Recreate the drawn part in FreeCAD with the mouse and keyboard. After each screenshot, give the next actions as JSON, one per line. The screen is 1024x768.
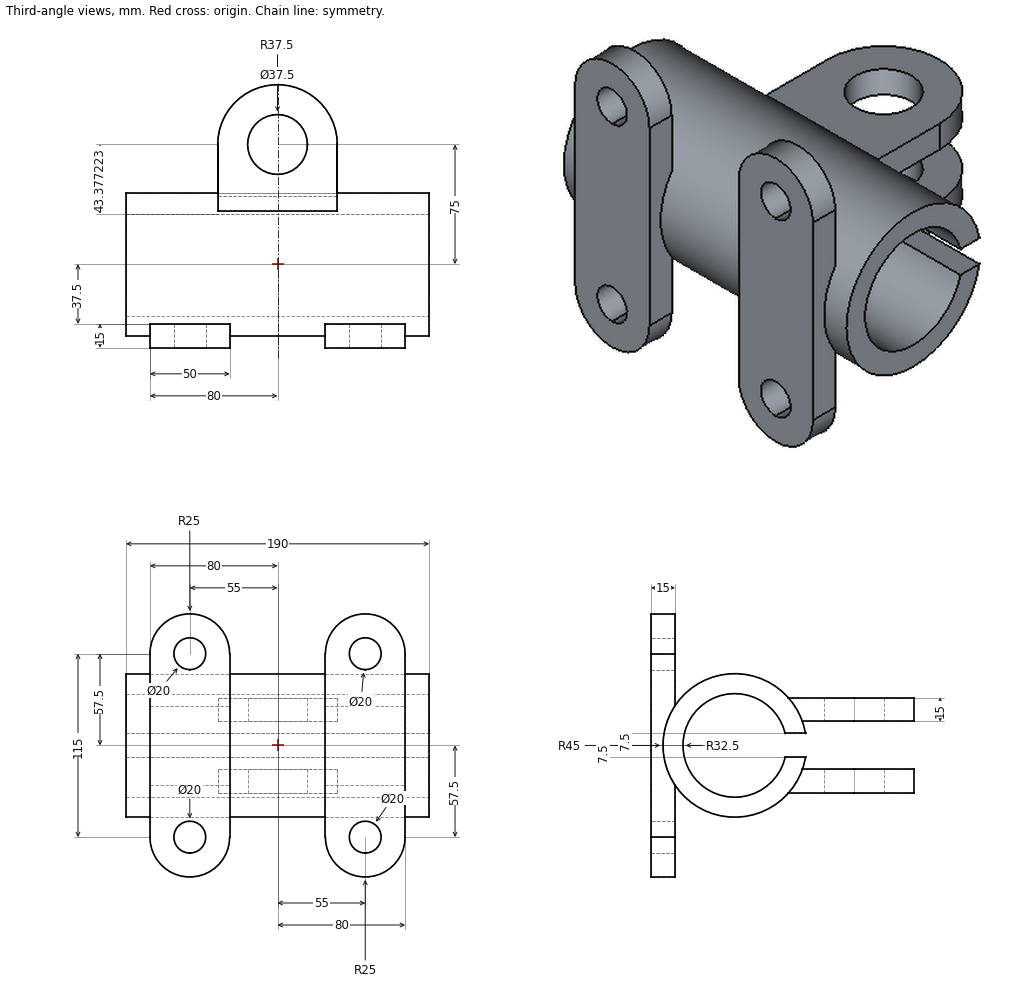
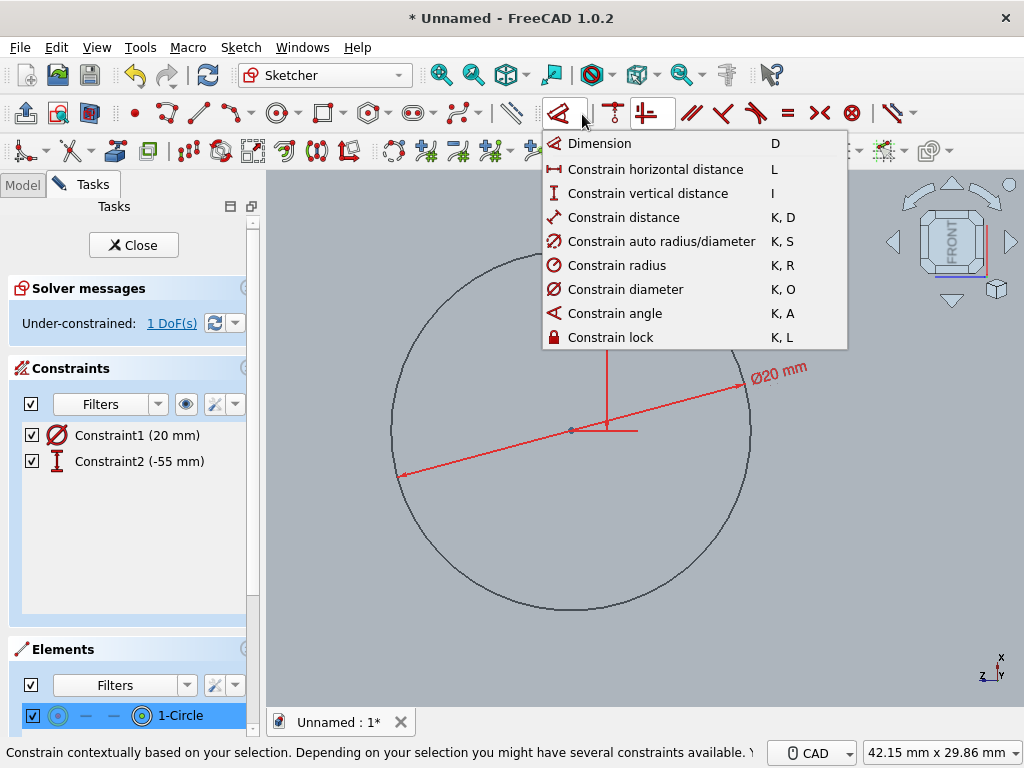
{"action": "left_click", "coordinate": [695, 169]}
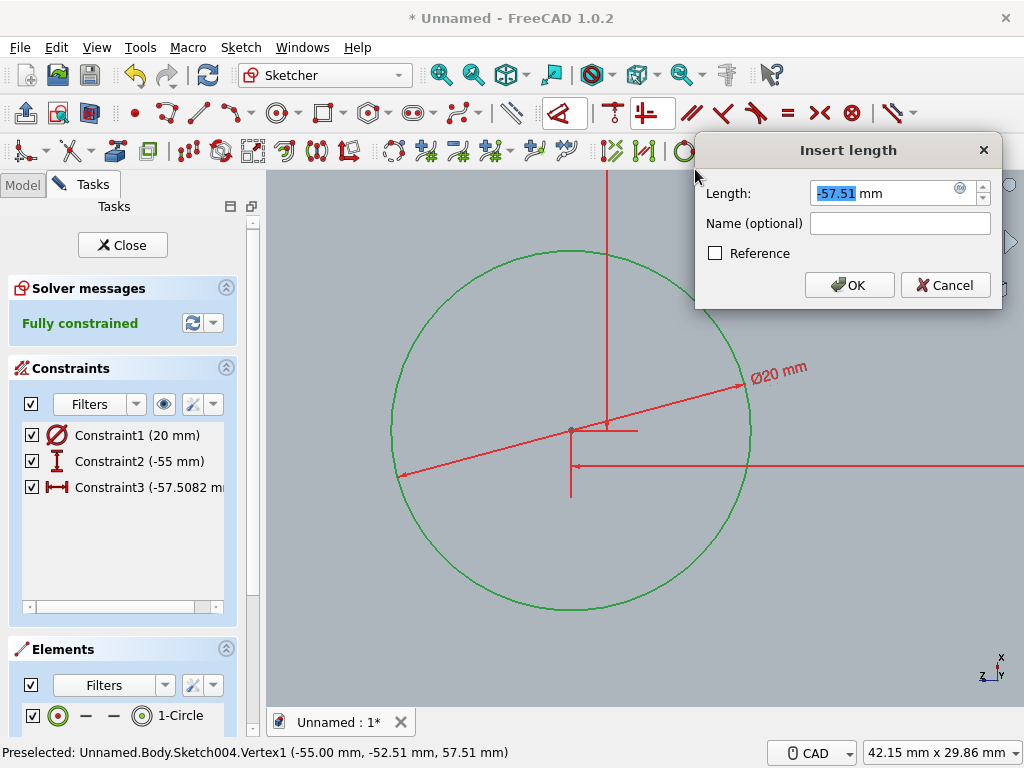
{"action": "type", "text": "-57.5"}
{"action": "key", "text": "Return"}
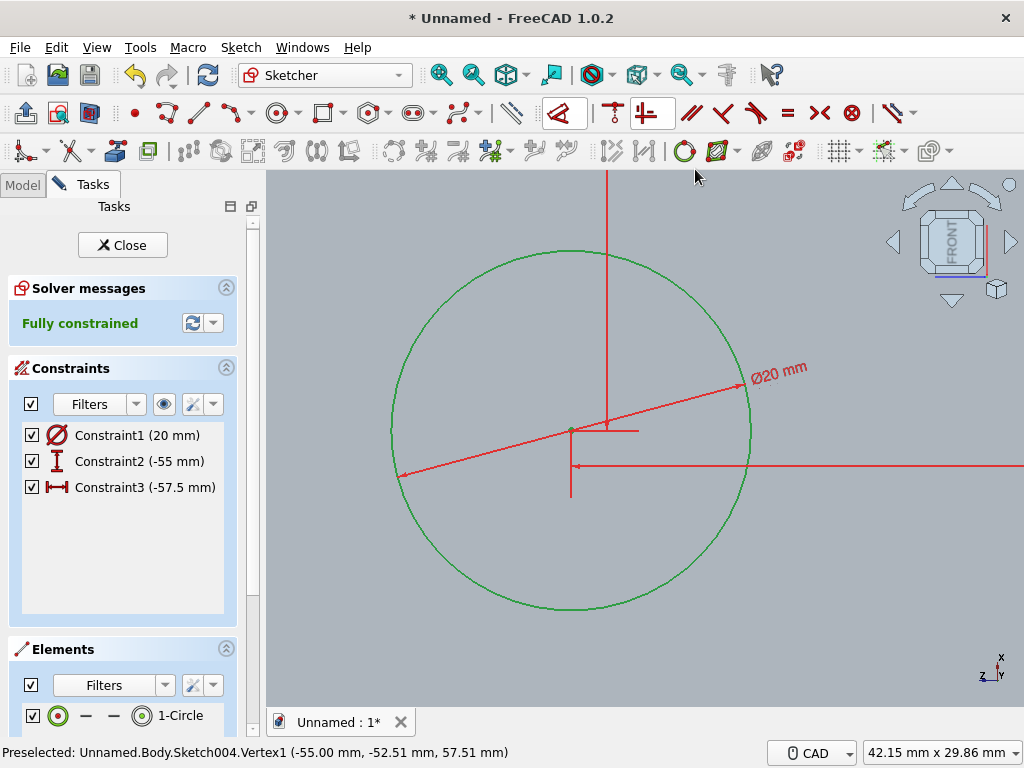
{"action": "left_click", "coordinate": [123, 245]}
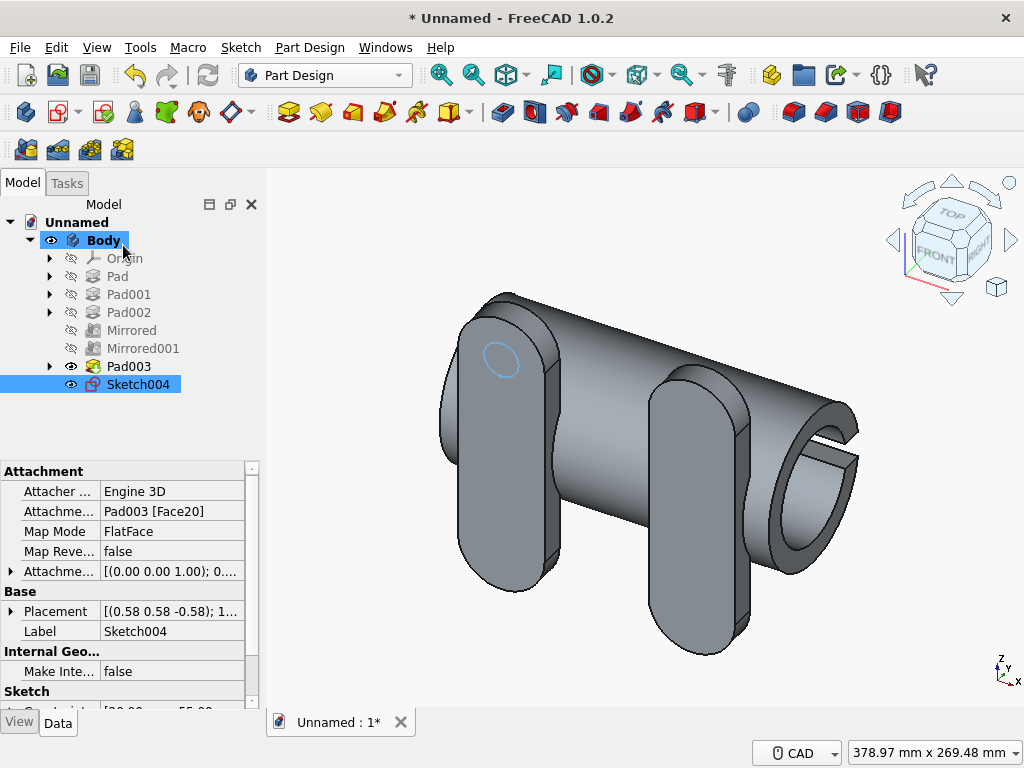
{"action": "left_click", "coordinate": [504, 112]}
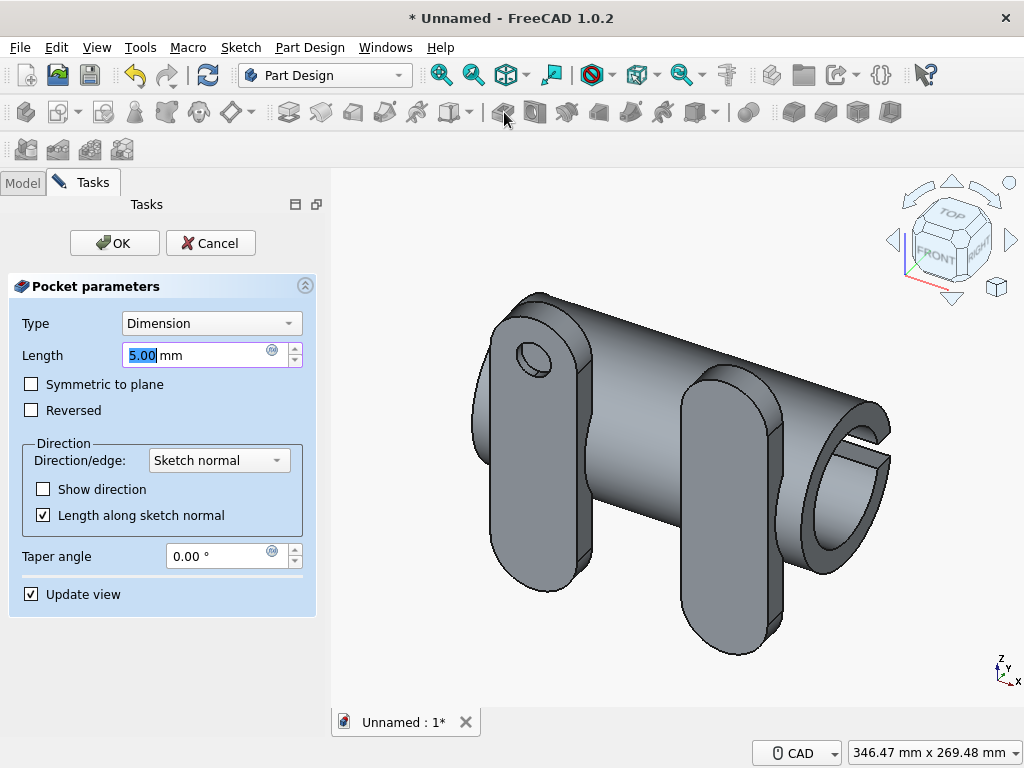
{"action": "left_click", "coordinate": [212, 324]}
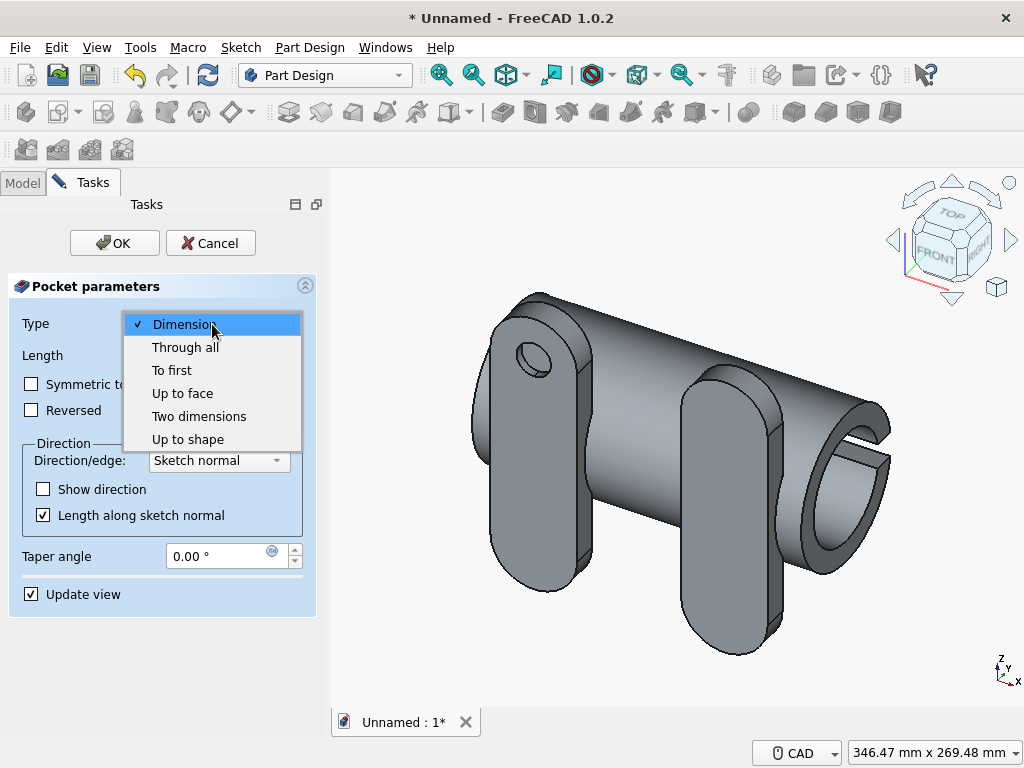
{"action": "left_click", "coordinate": [212, 370]}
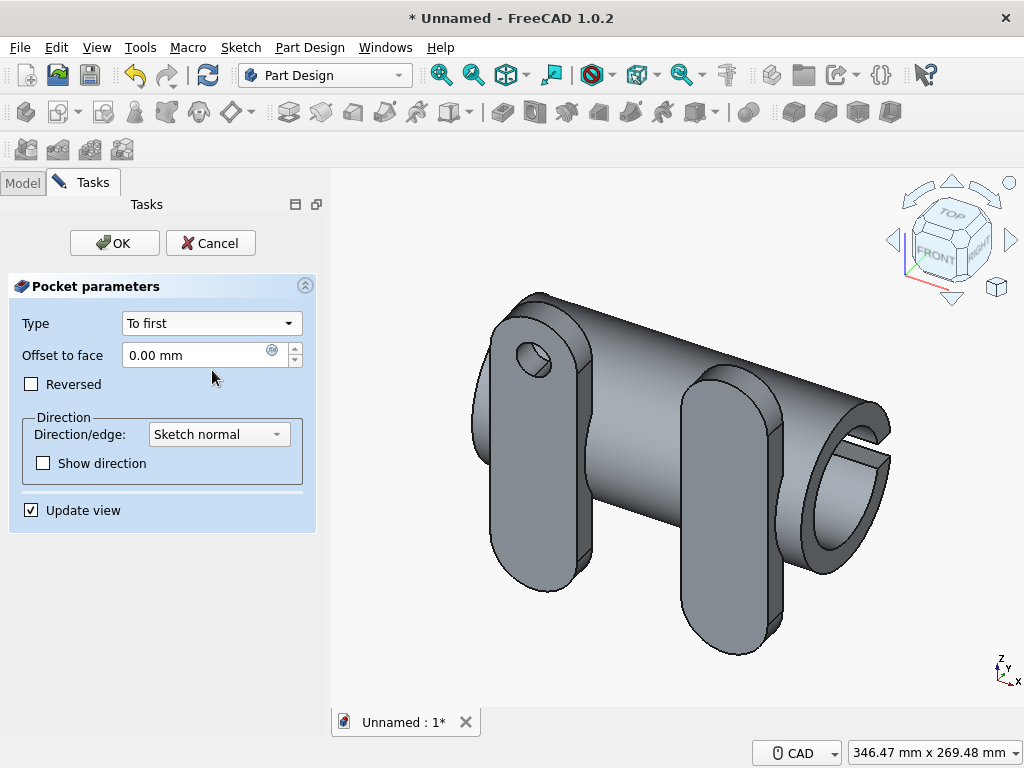
{"action": "left_click", "coordinate": [115, 243]}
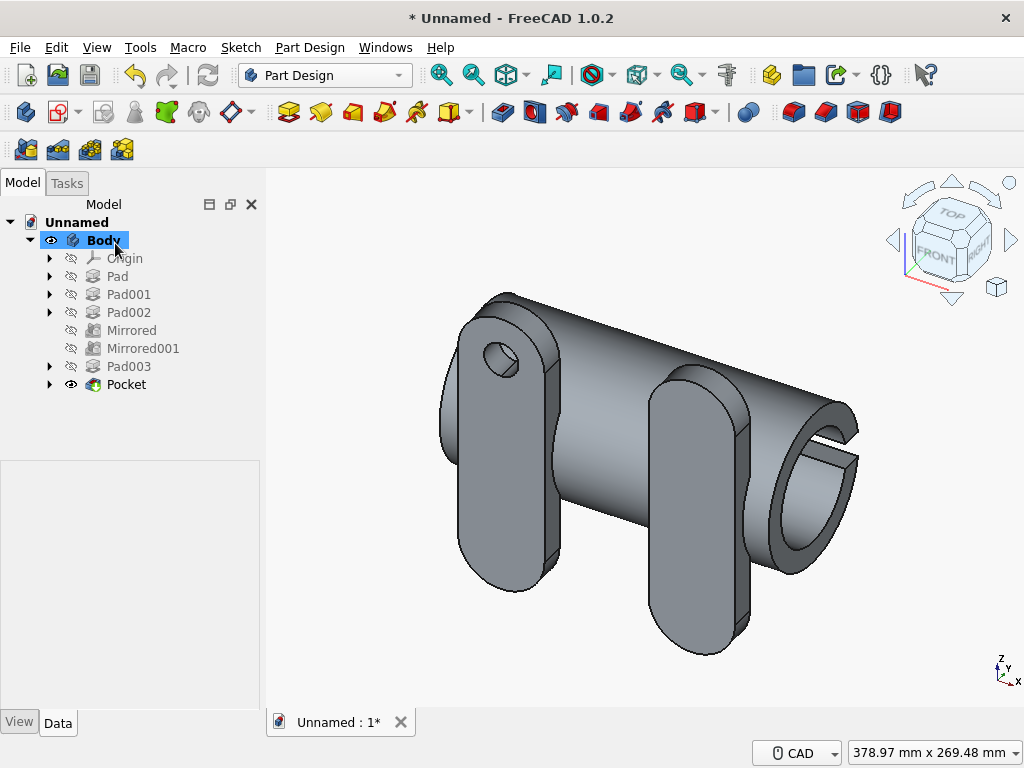
{"action": "left_click", "coordinate": [692, 516]}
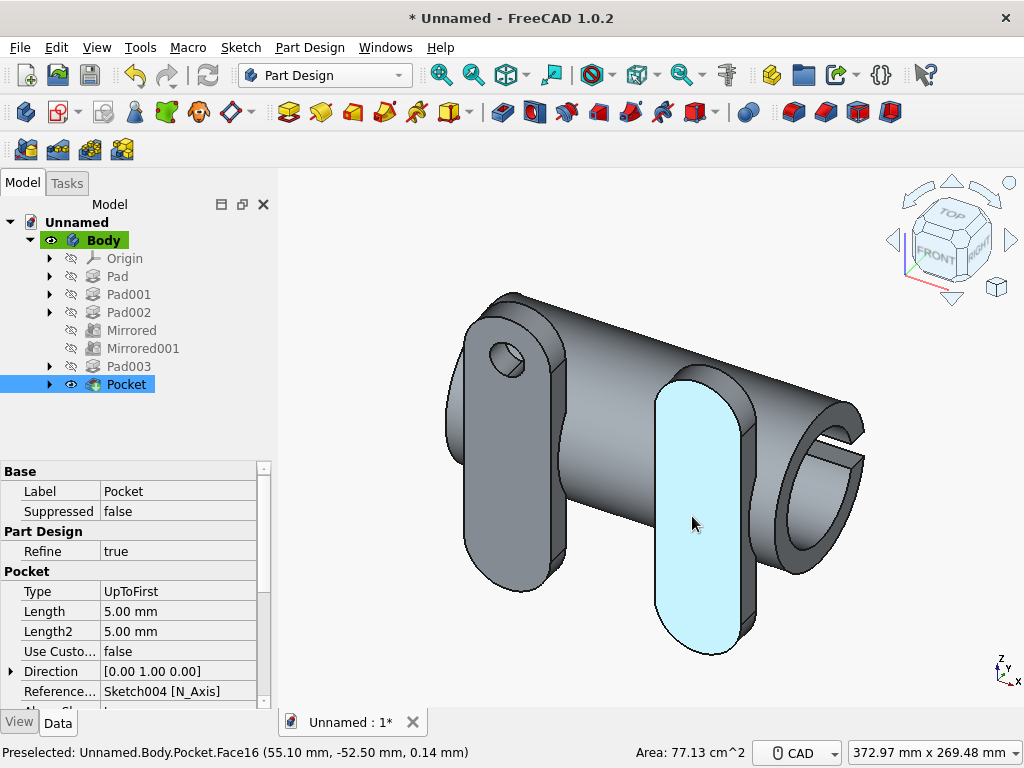
{"action": "left_click", "coordinate": [58, 112]}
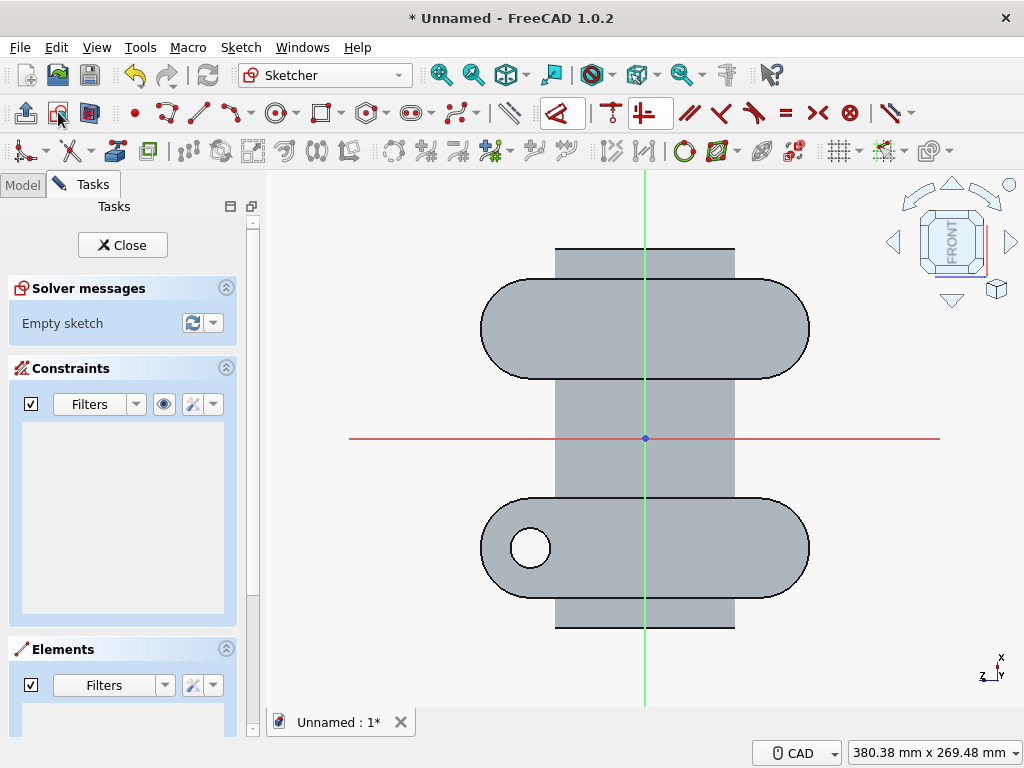
{"action": "scroll", "coordinate": [782, 562], "scroll_direction": "up", "scroll_amount": 11}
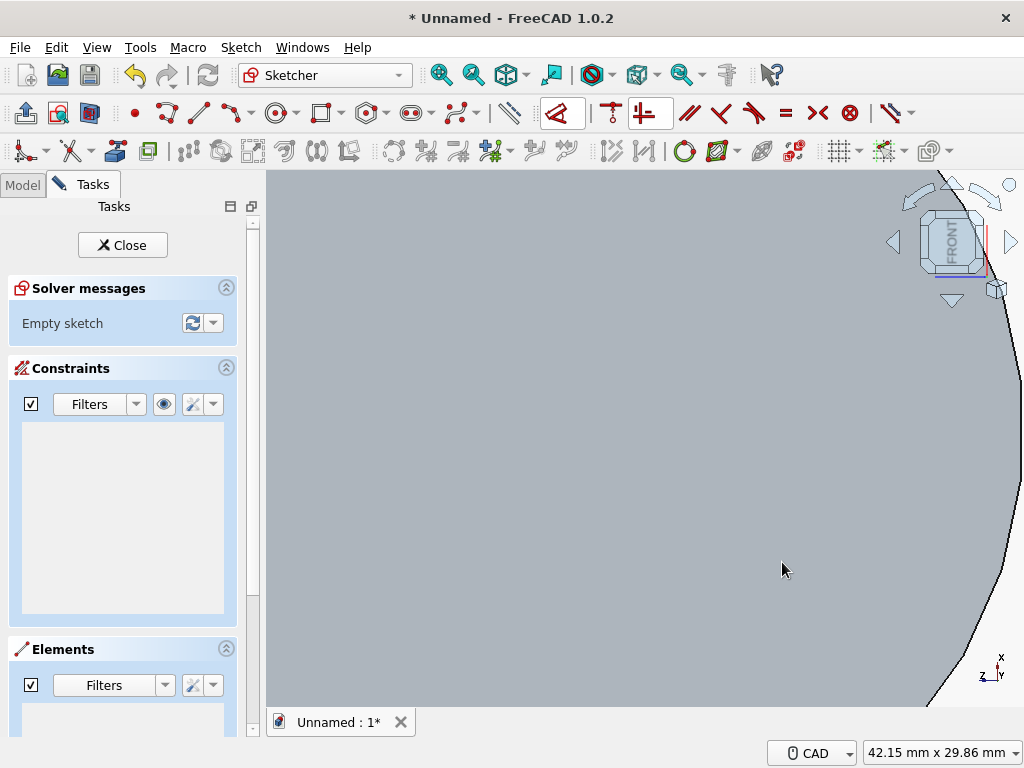
{"action": "left_click", "coordinate": [276, 114]}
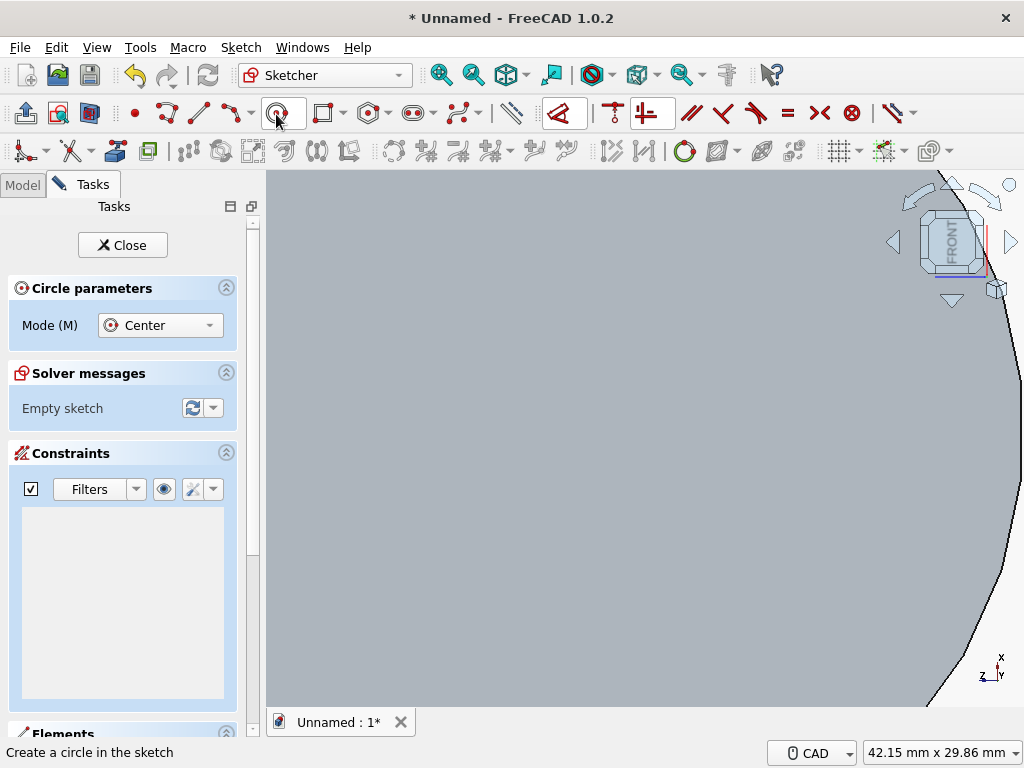
{"action": "left_click", "coordinate": [574, 431]}
{"action": "left_click", "coordinate": [701, 304]}
{"action": "key", "text": "Escape"}